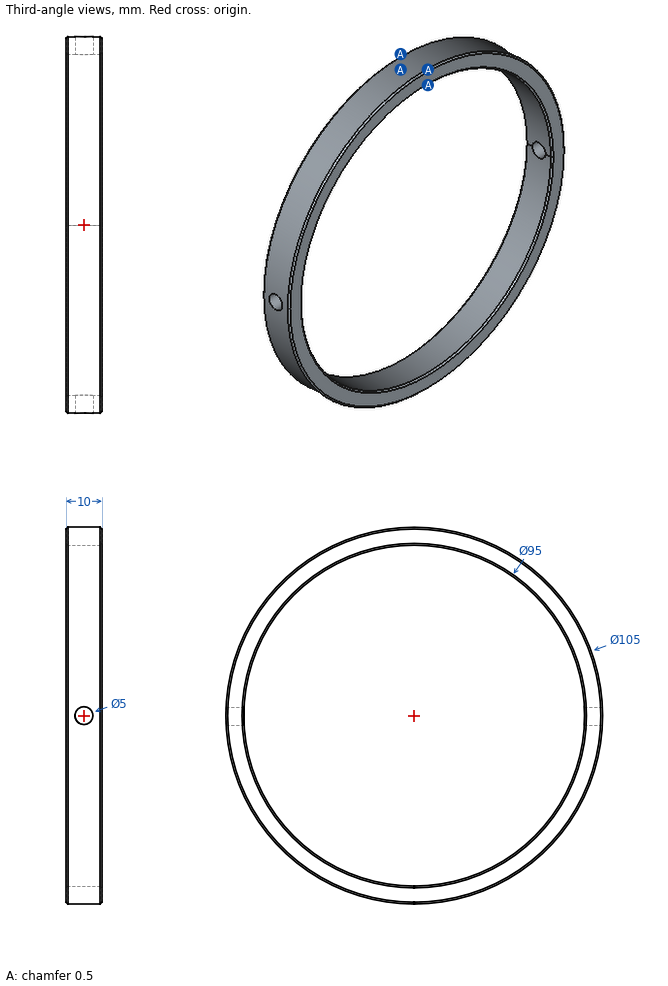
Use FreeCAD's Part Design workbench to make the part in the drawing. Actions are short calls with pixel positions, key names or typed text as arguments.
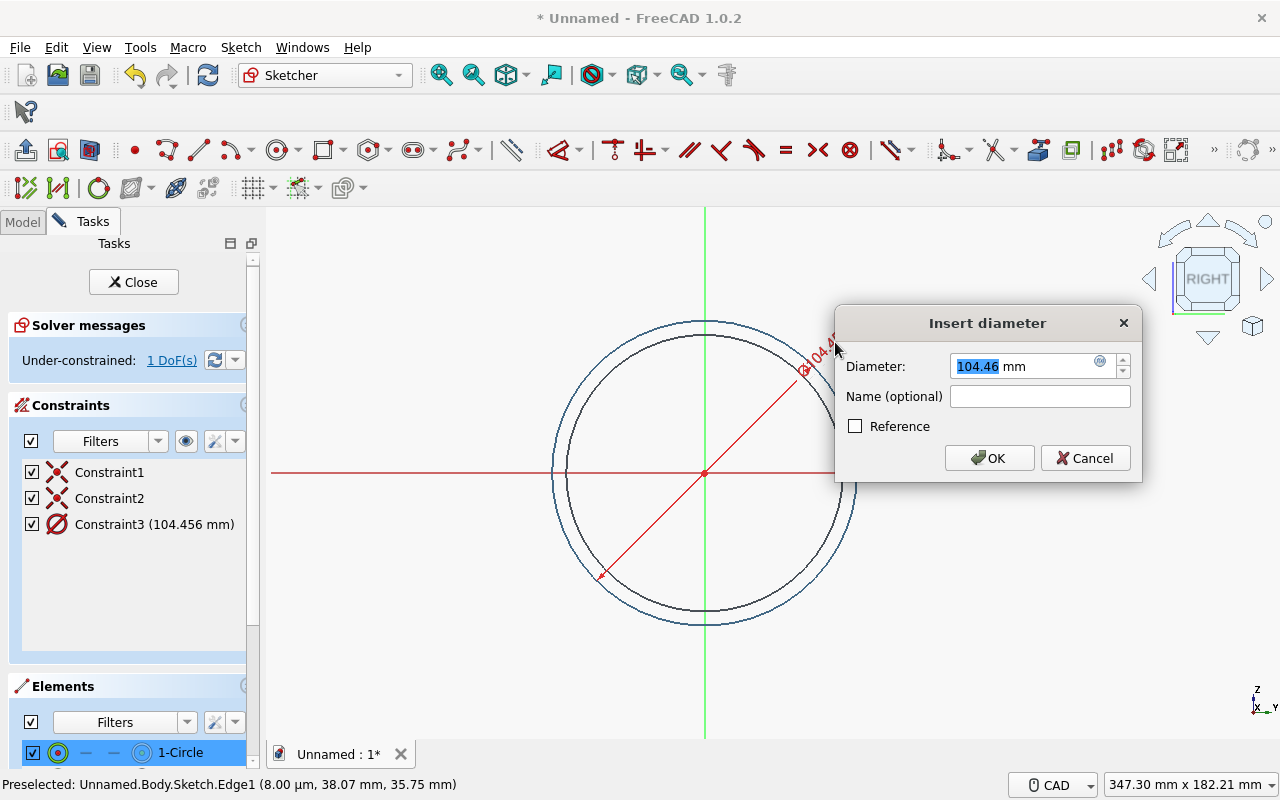
text(105)
key(Return)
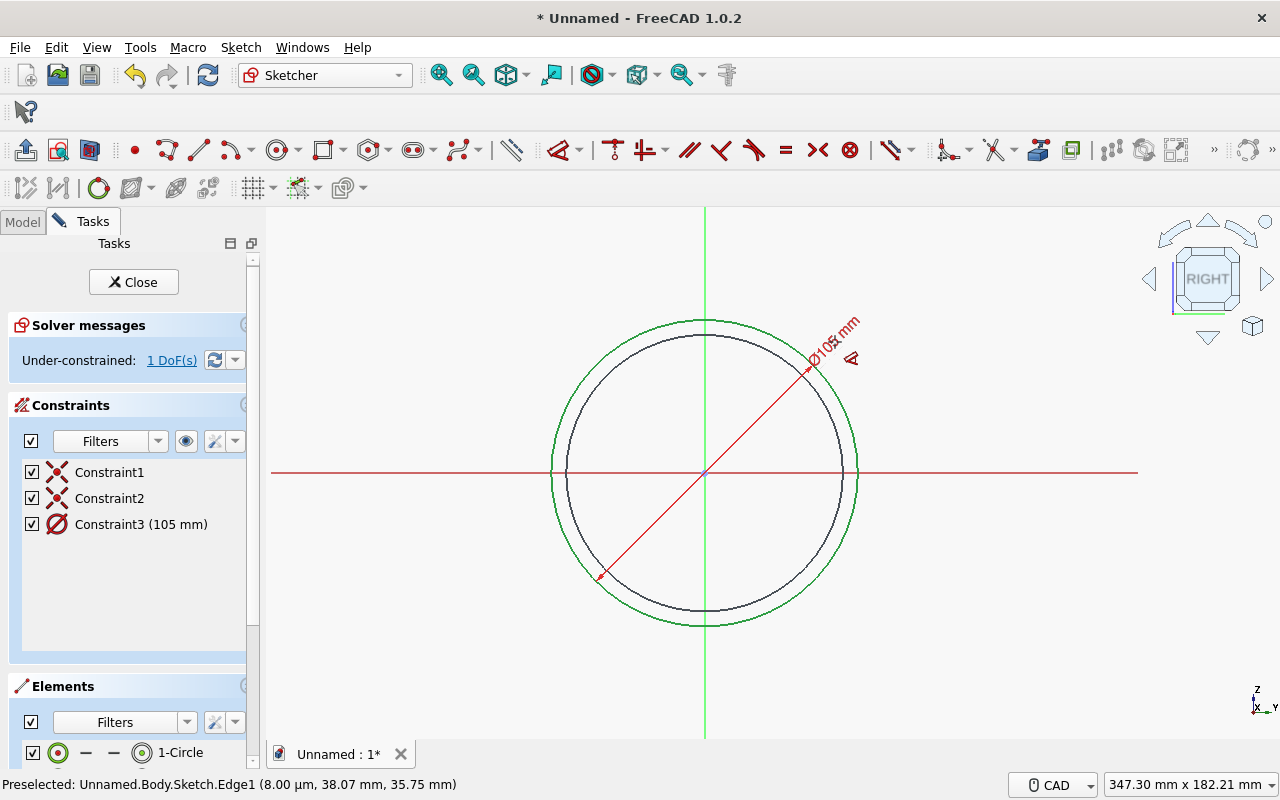
click(802, 375)
click(868, 425)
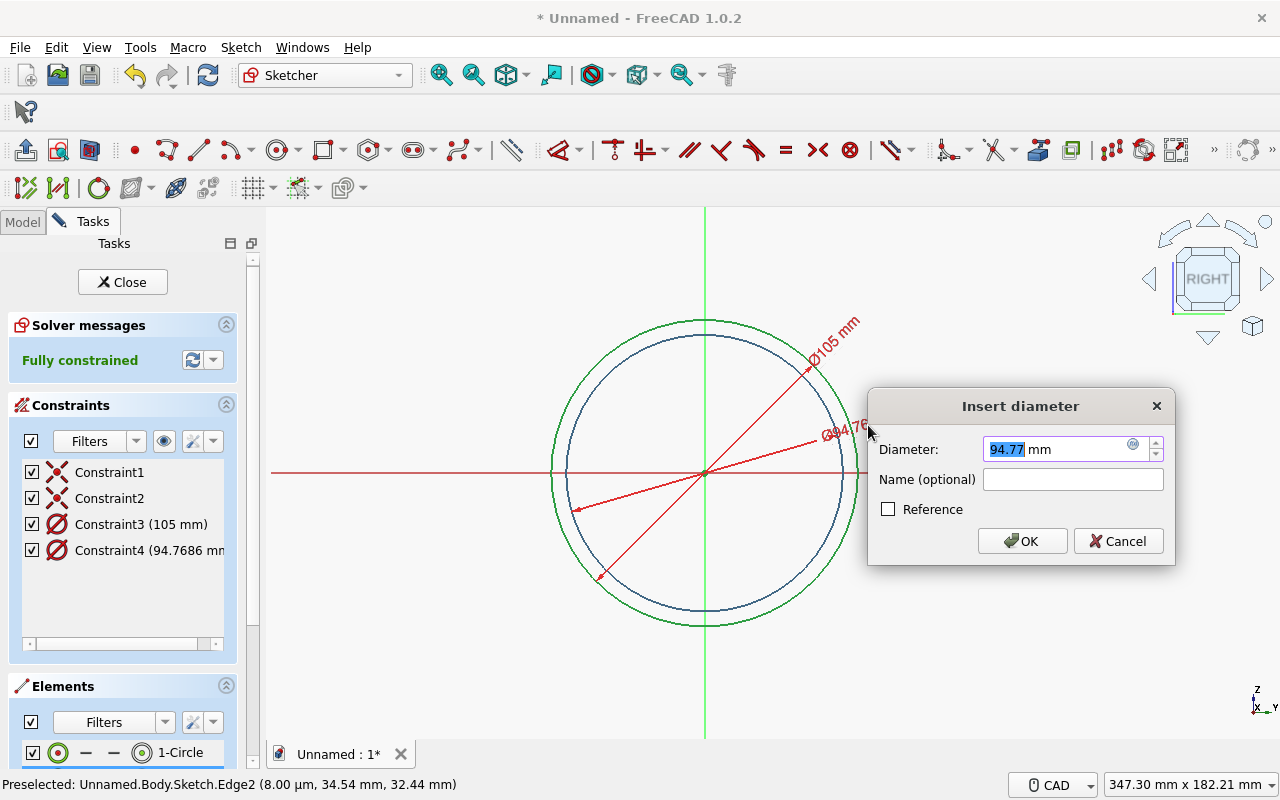
text(95)
key(Return)
key(Escape)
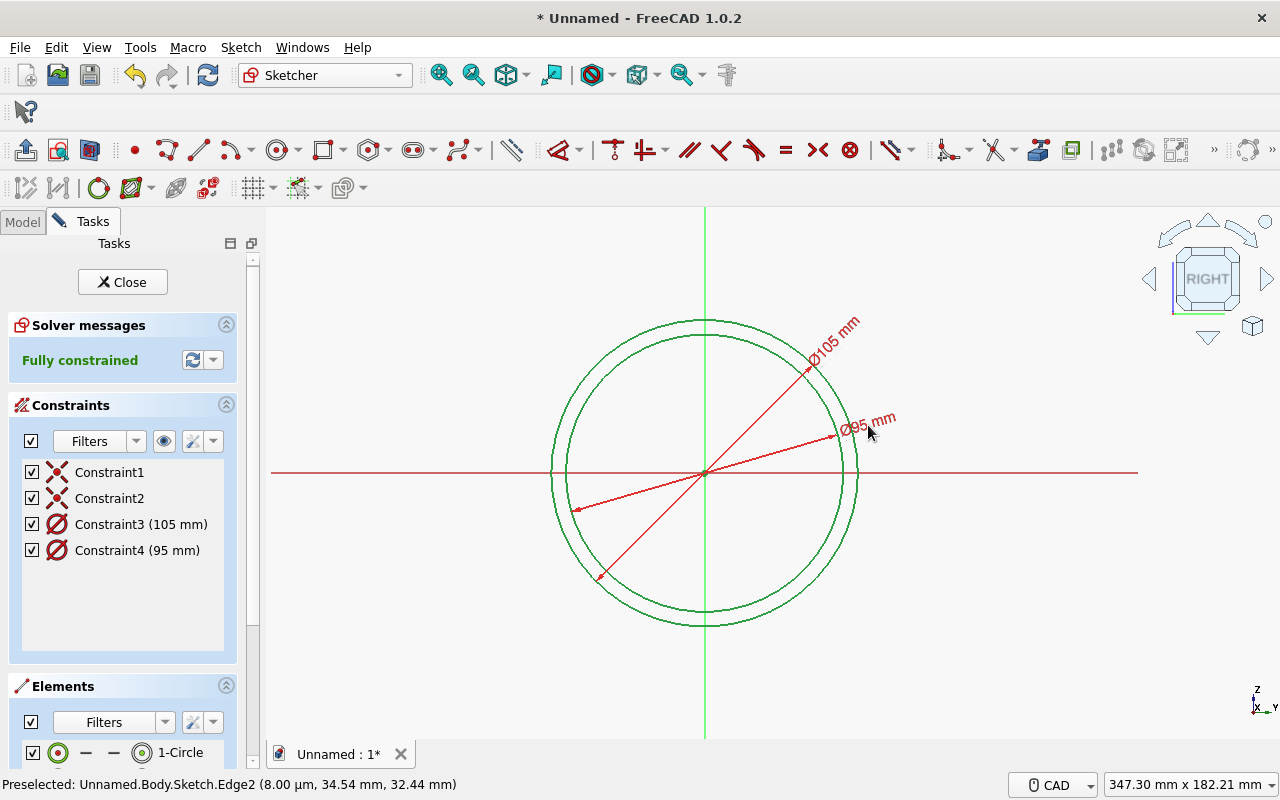
click(123, 282)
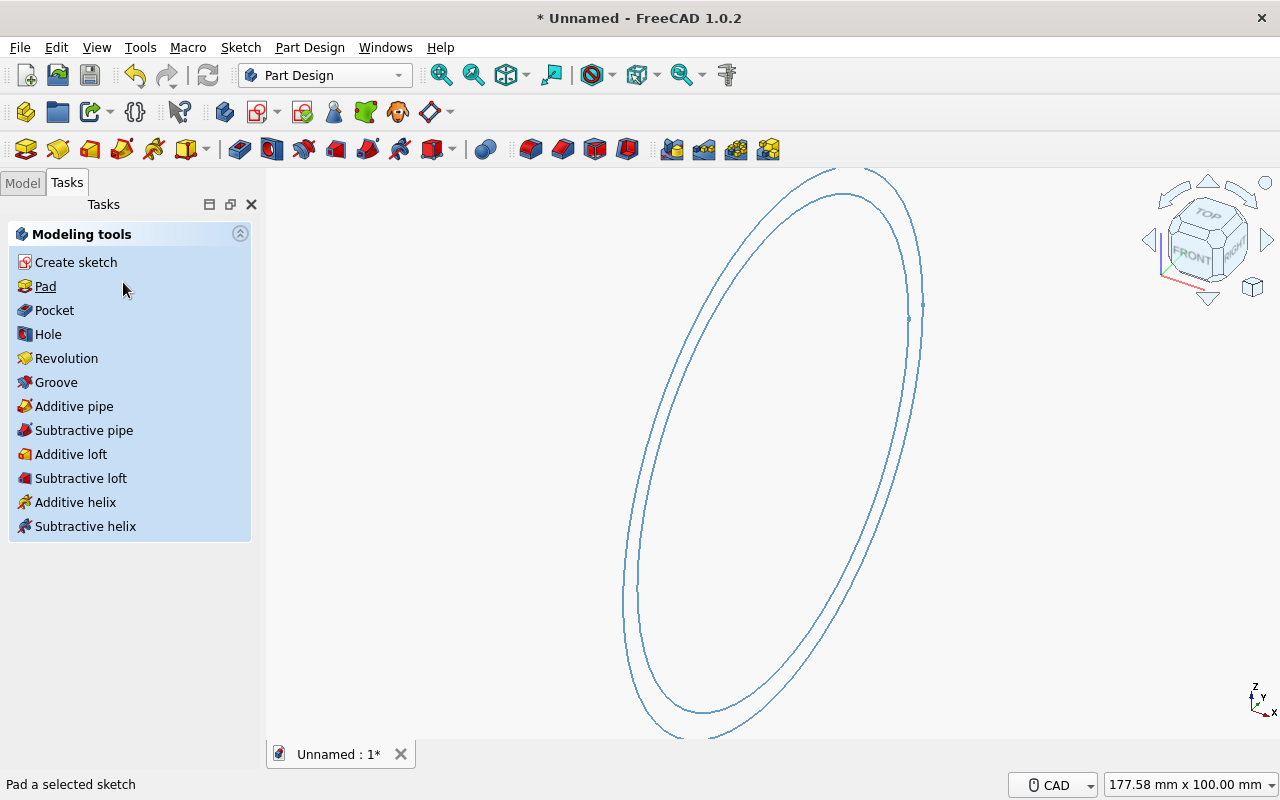
click(26, 150)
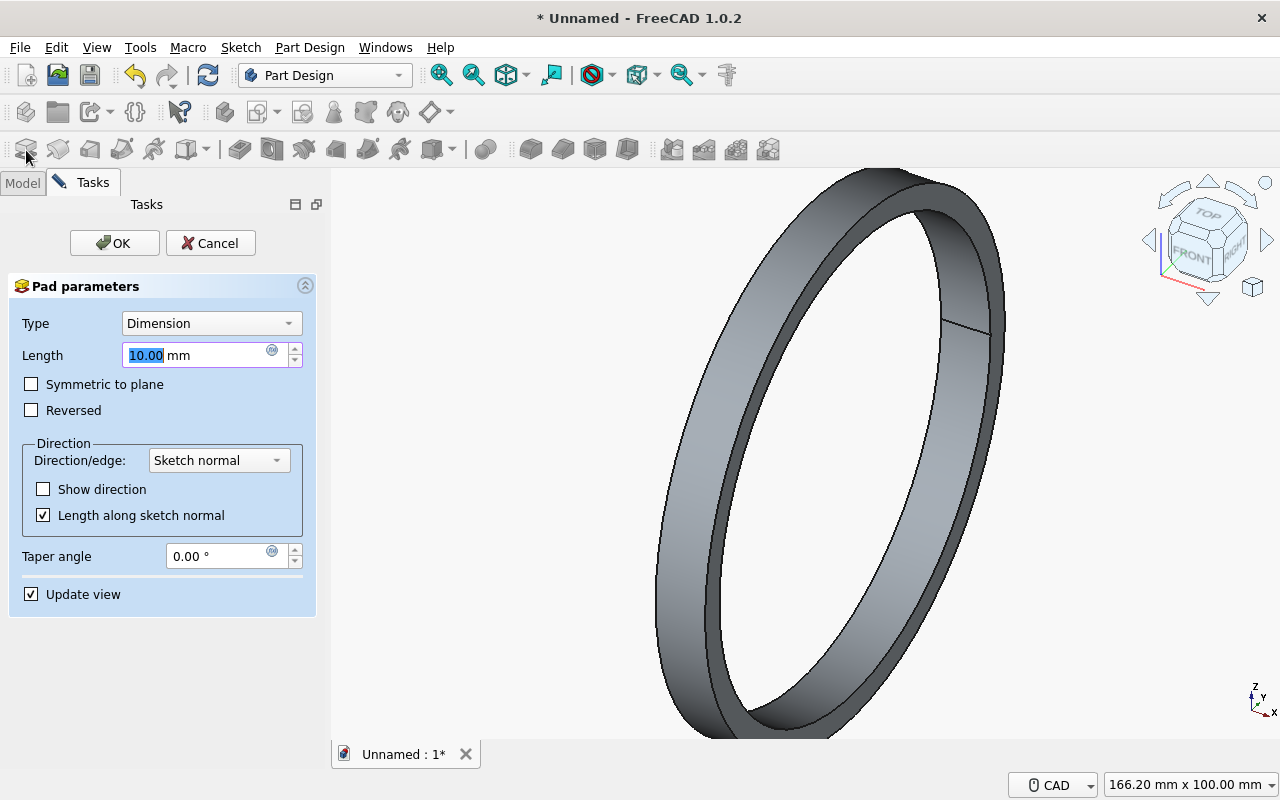
text(10)
key(Tab)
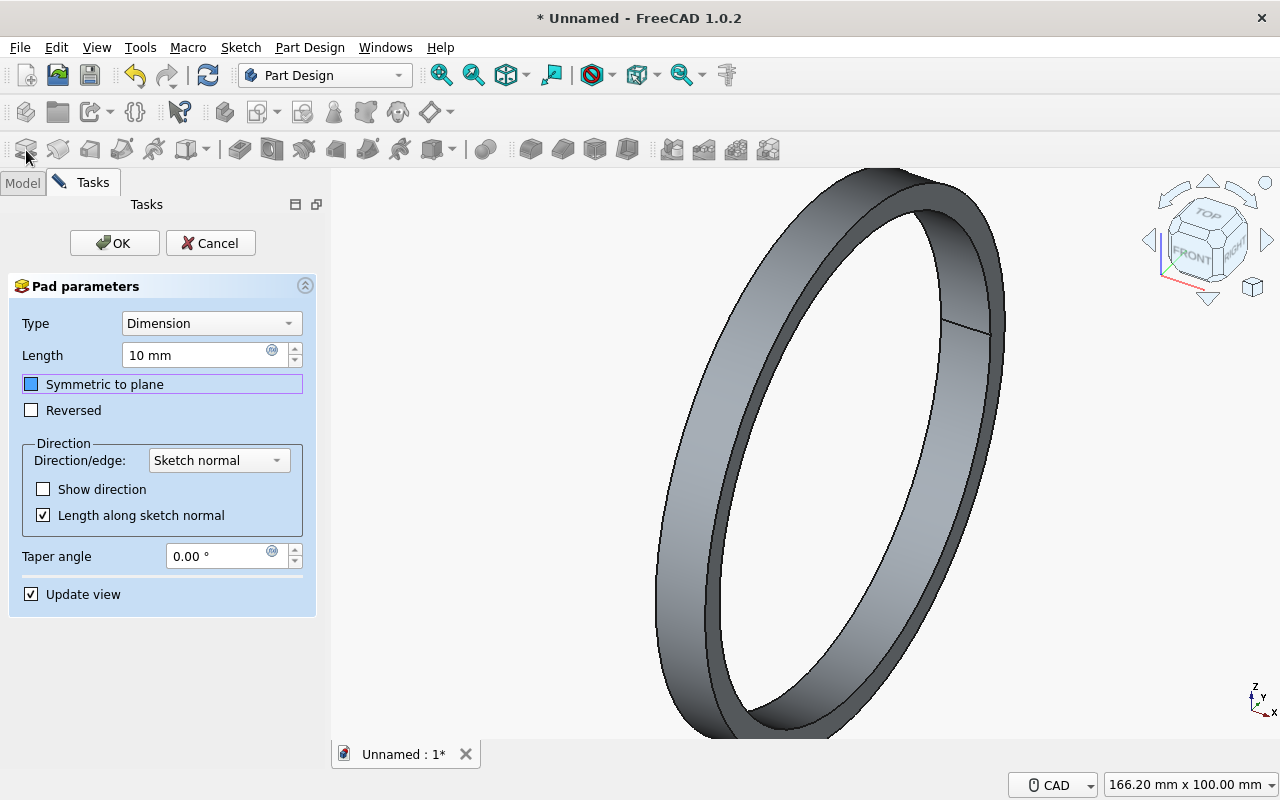
click(30, 384)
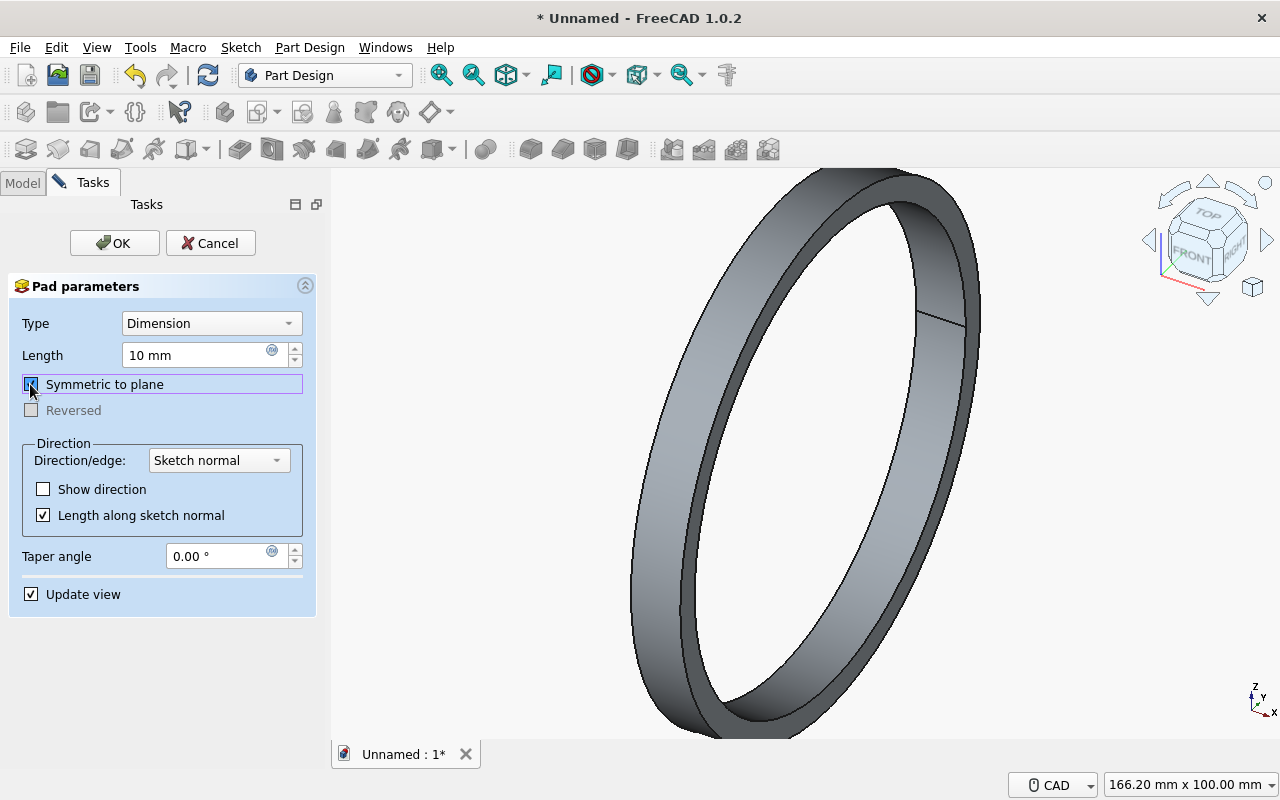
click(115, 243)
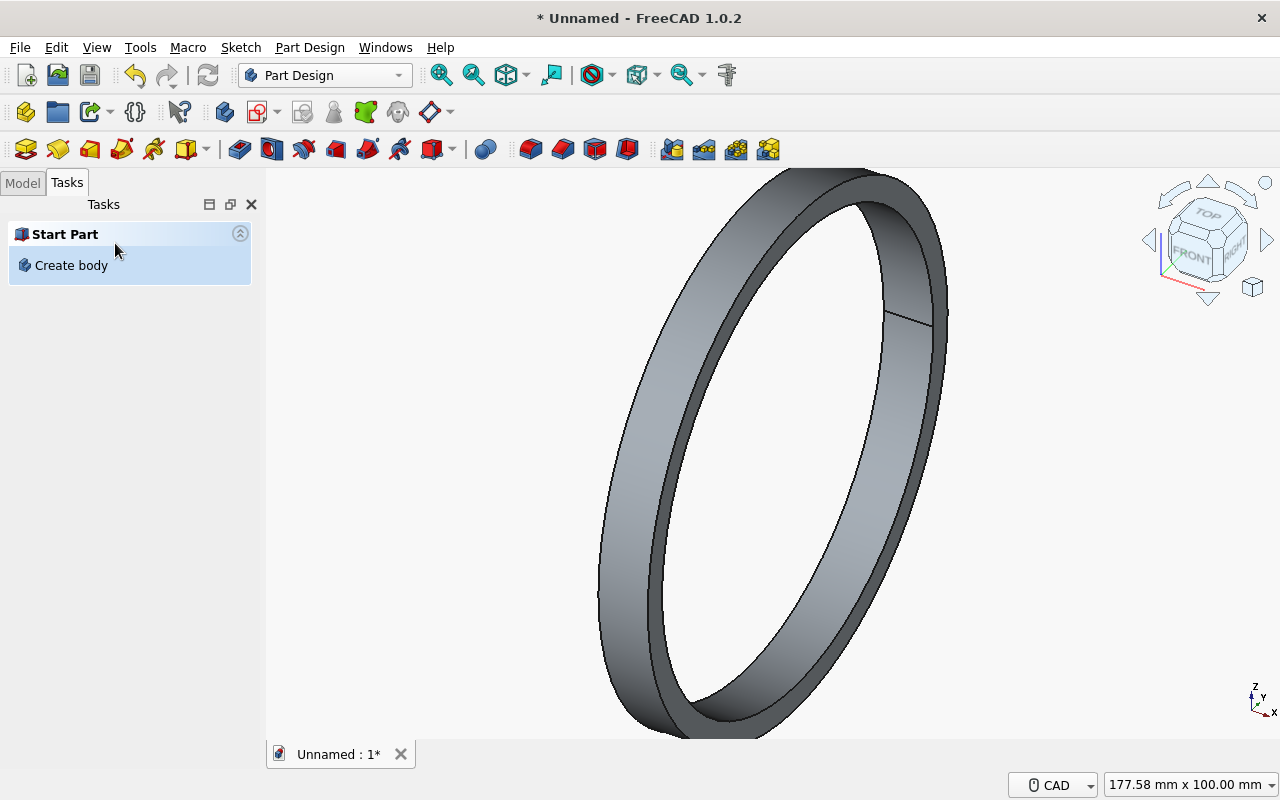
click(442, 76)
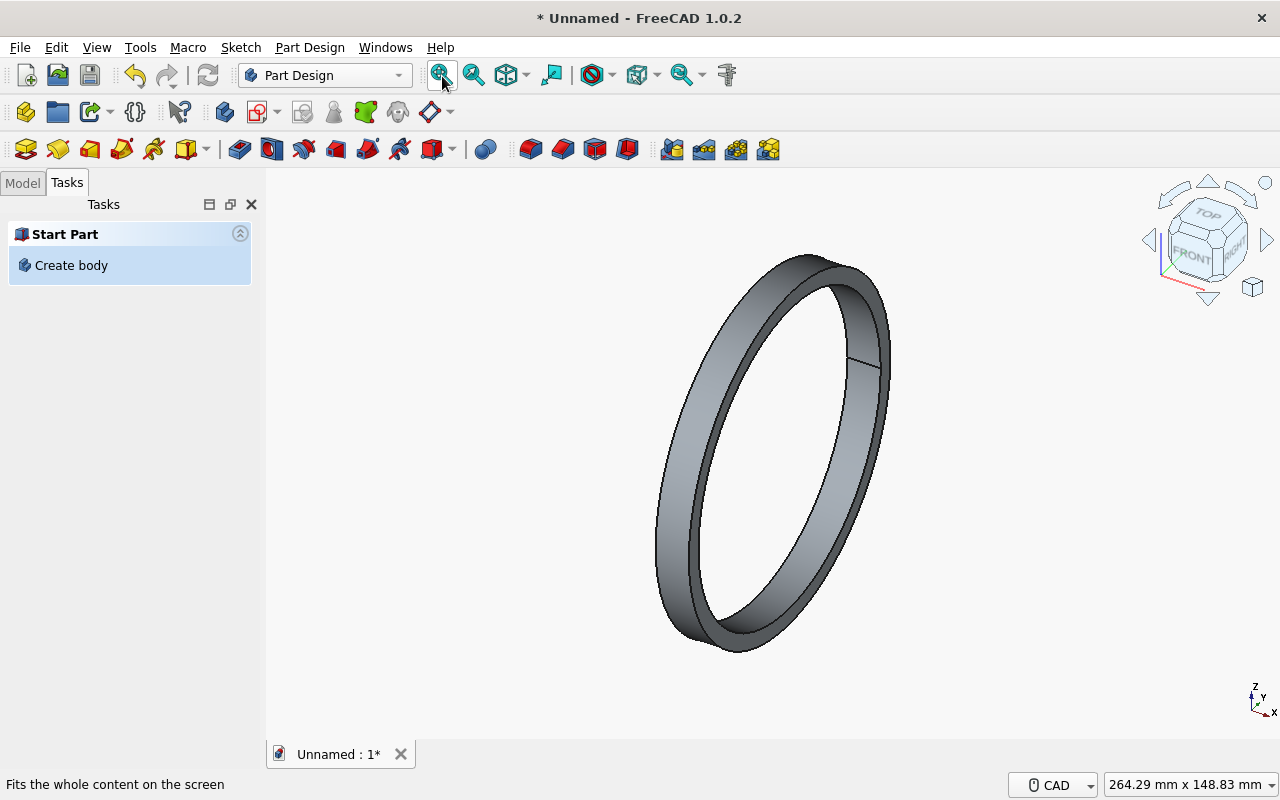
click(689, 558)